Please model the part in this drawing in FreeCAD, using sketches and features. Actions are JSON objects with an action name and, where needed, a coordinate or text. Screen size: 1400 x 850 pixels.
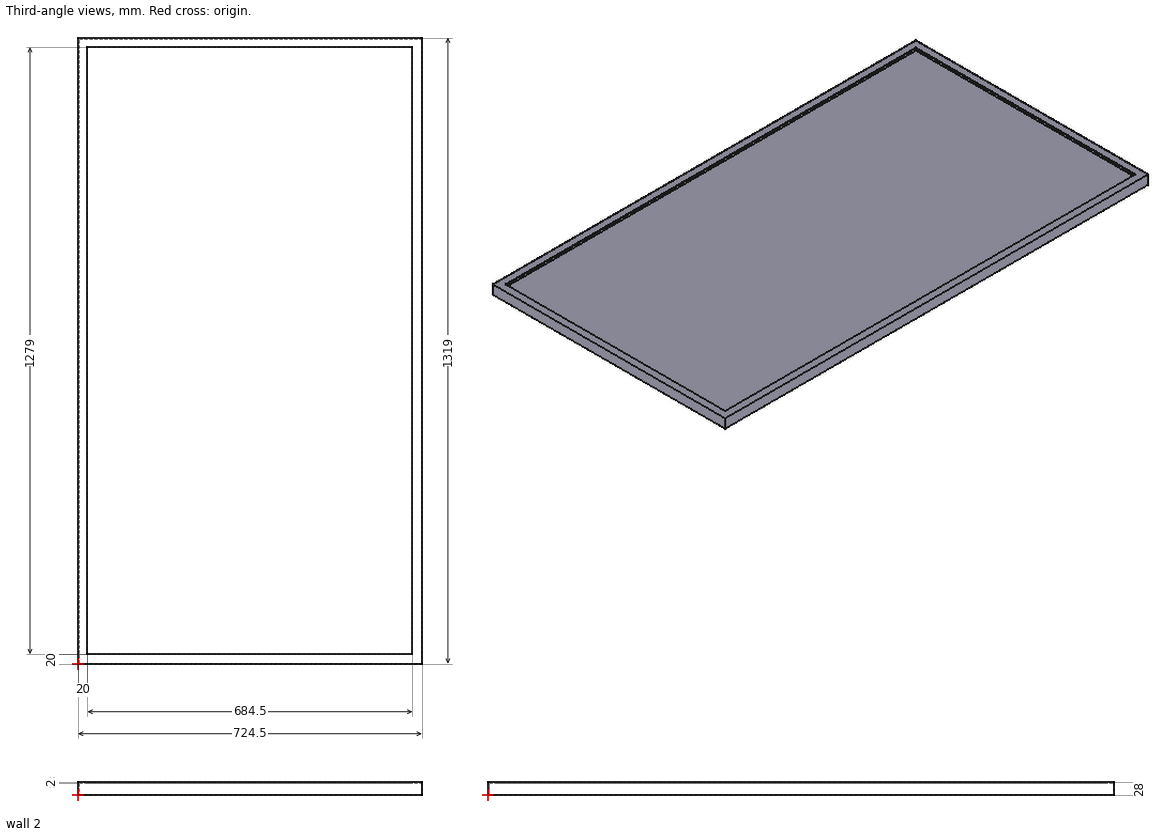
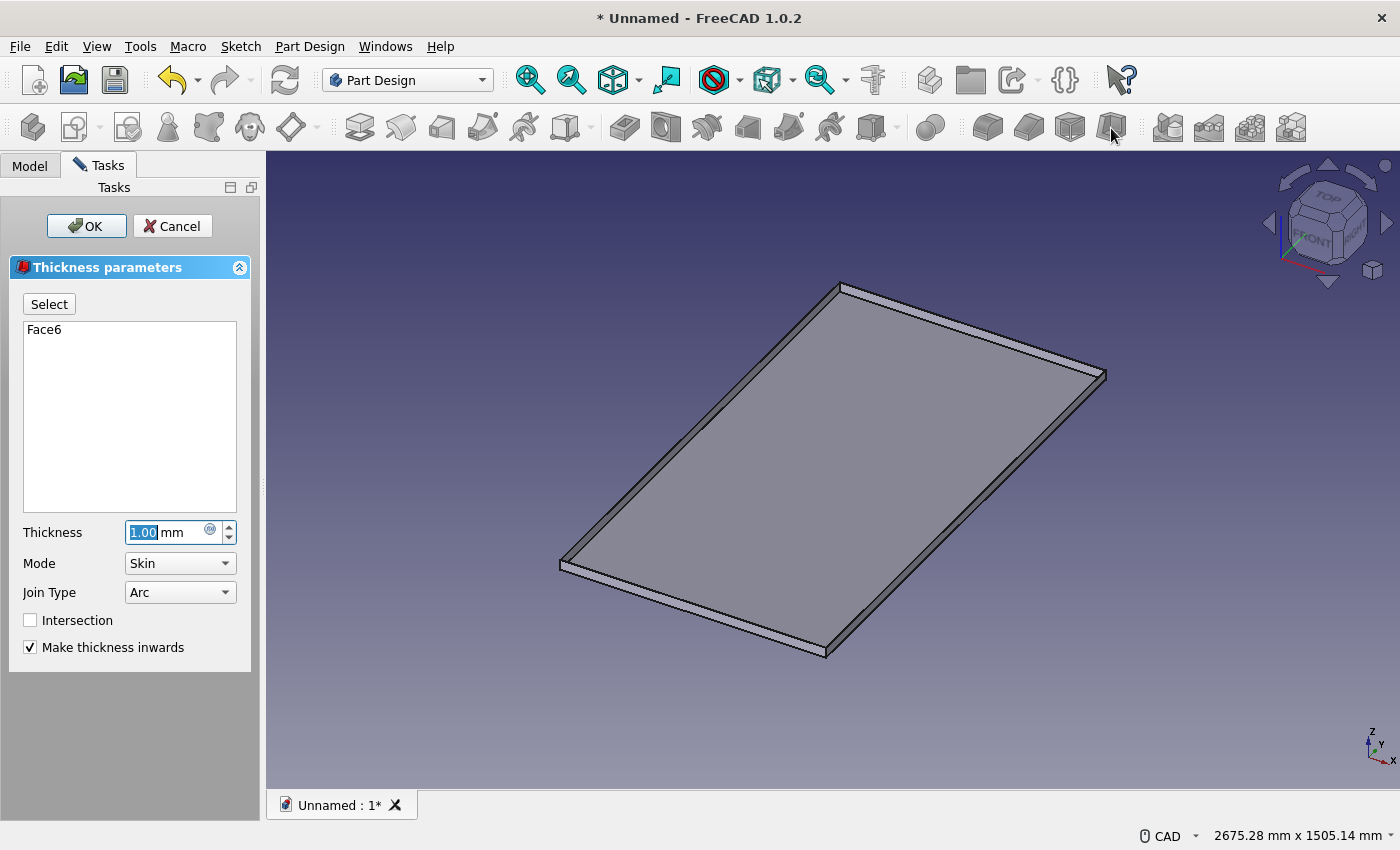
{"action": "type", "text": "2"}
{"action": "key", "text": "Tab"}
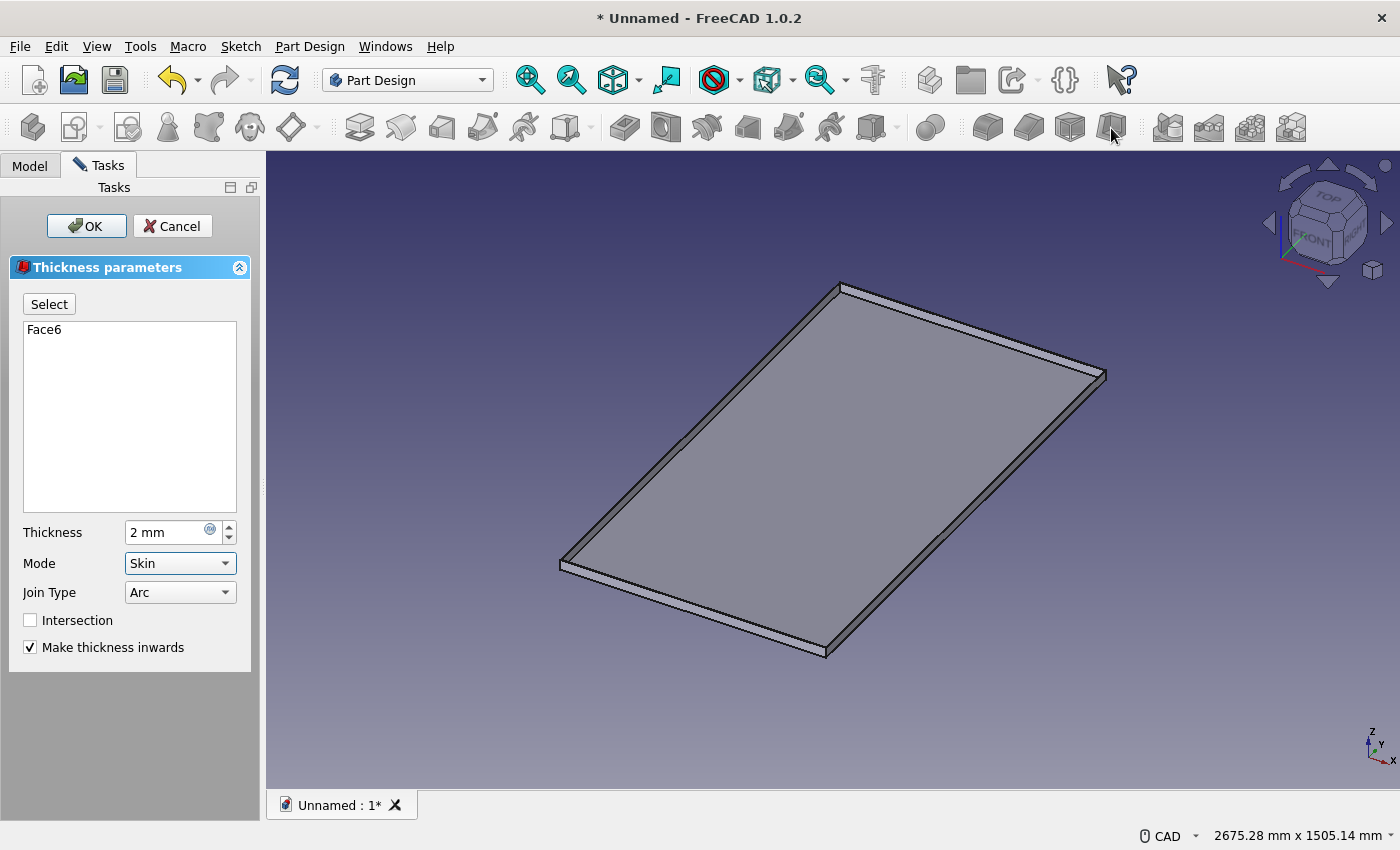
{"action": "left_click", "coordinate": [181, 592]}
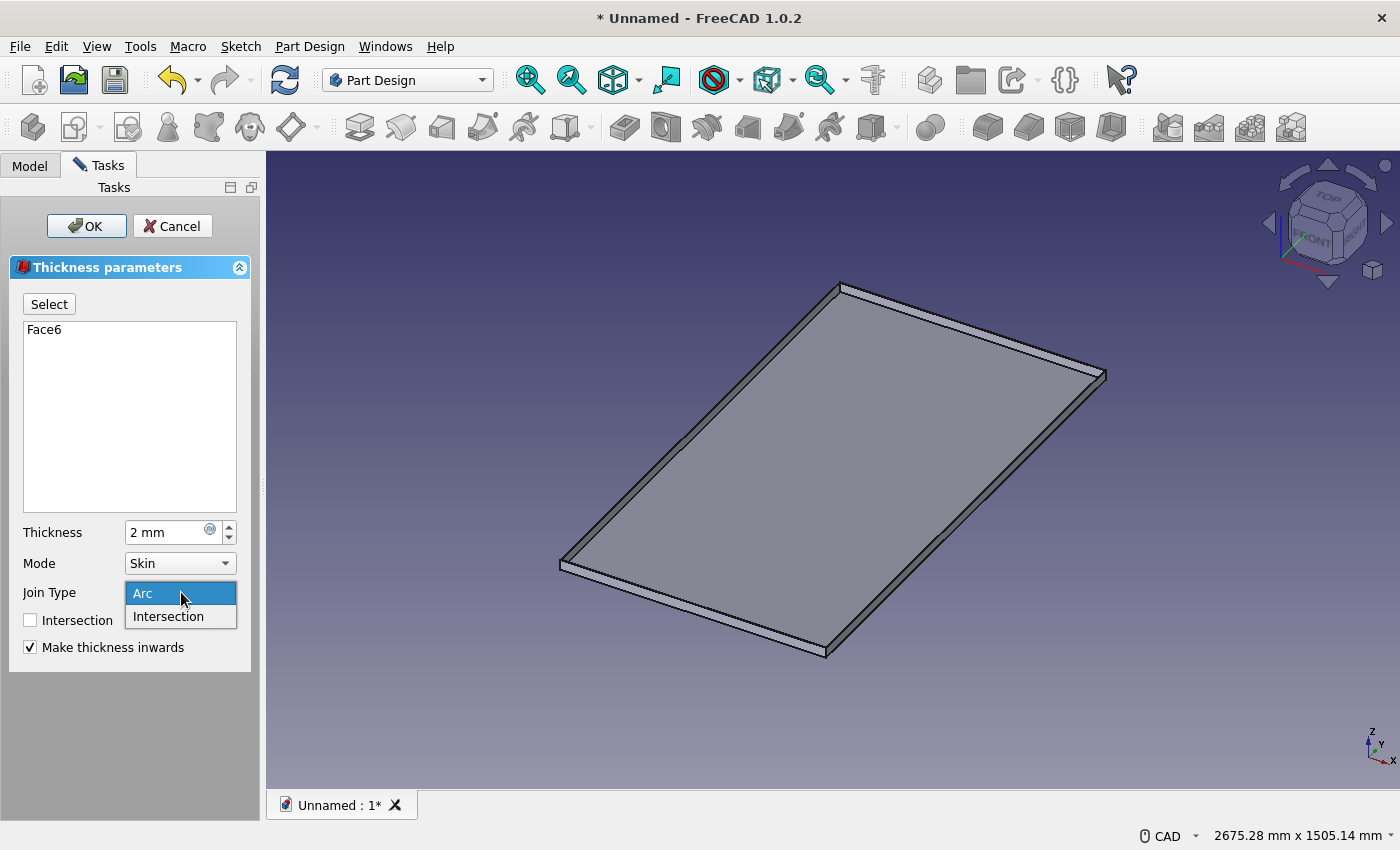
{"action": "left_click", "coordinate": [179, 616]}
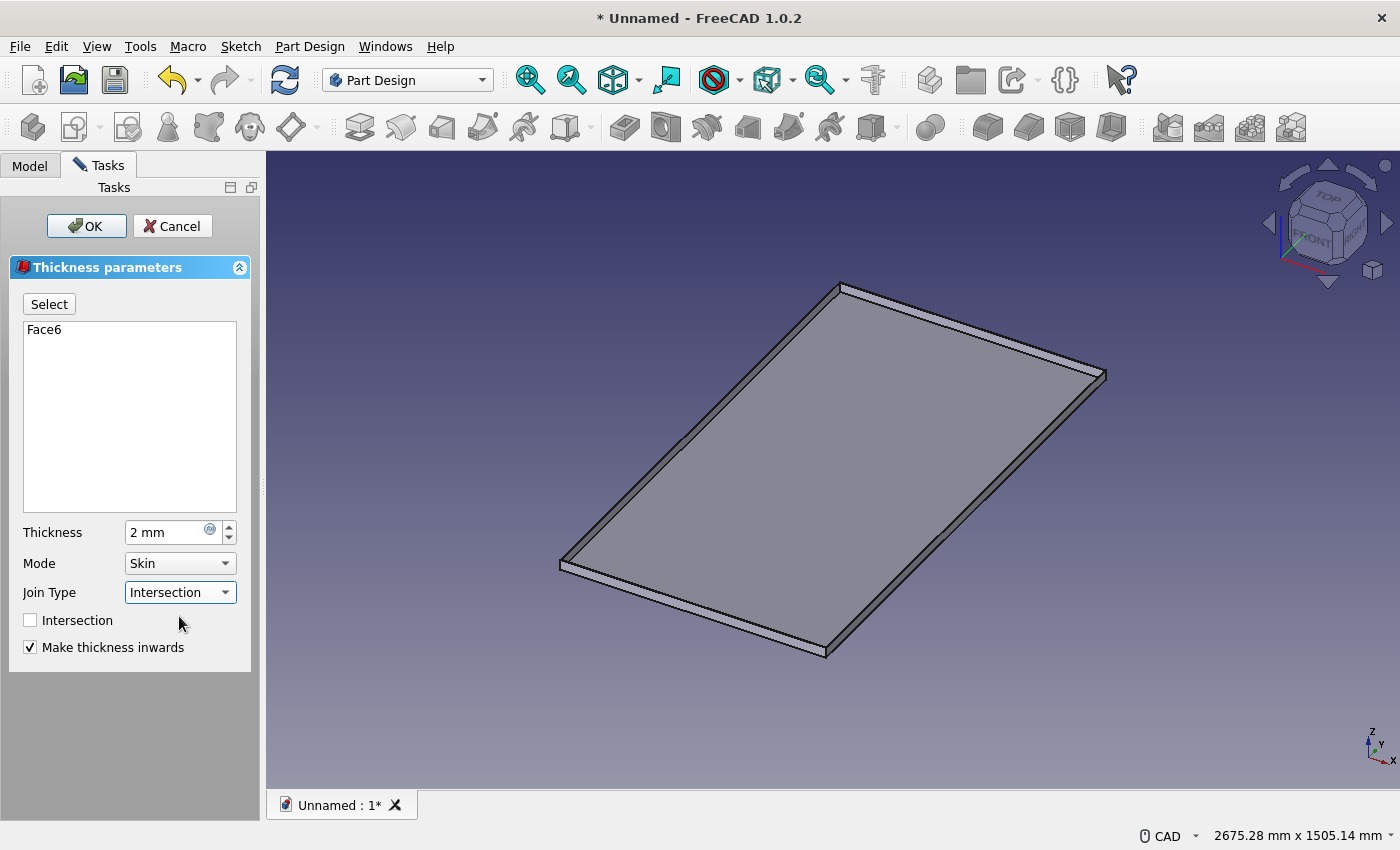
{"action": "left_click", "coordinate": [87, 226]}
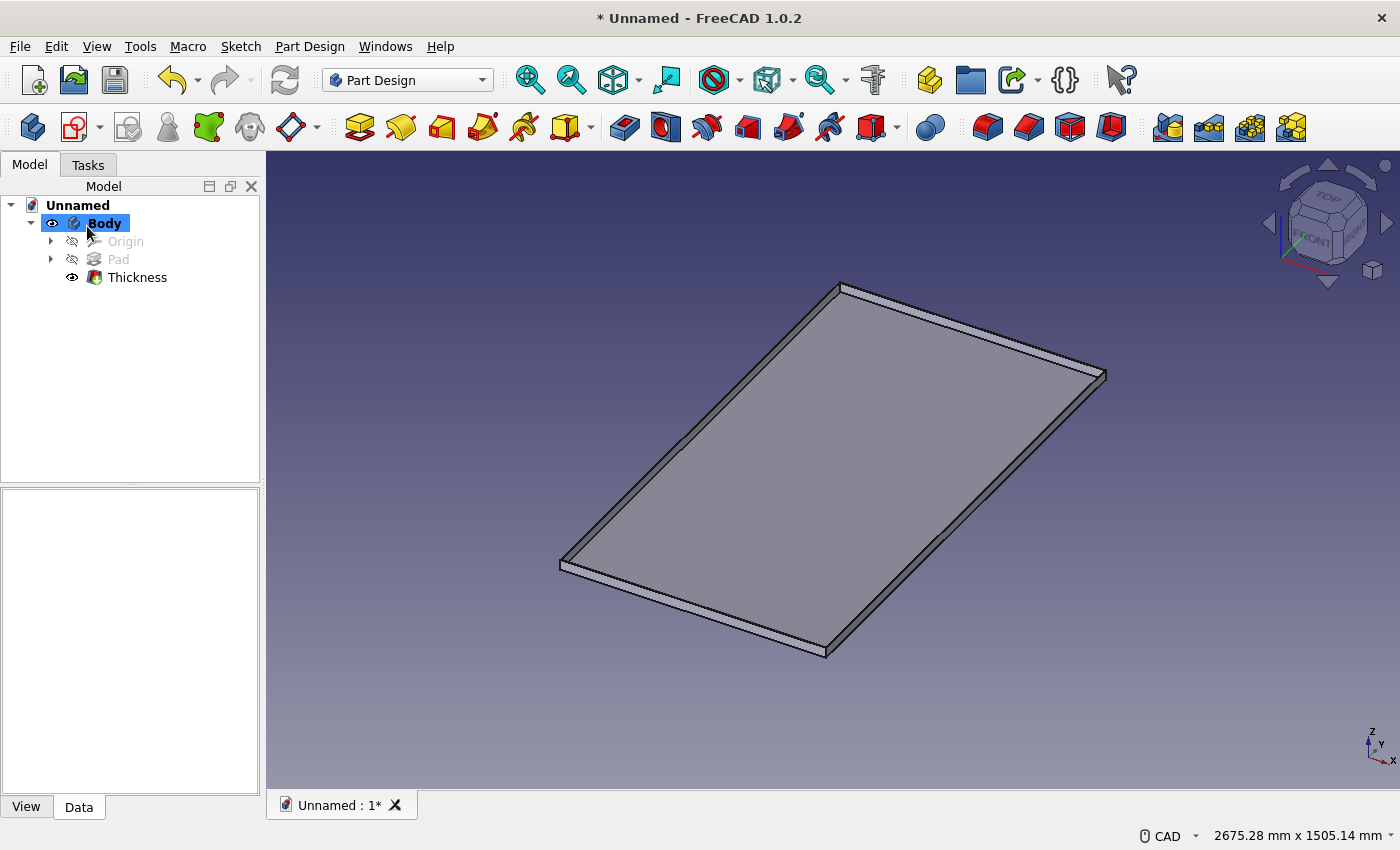
{"action": "scroll", "coordinate": [1017, 340], "scroll_direction": "up", "scroll_amount": 15}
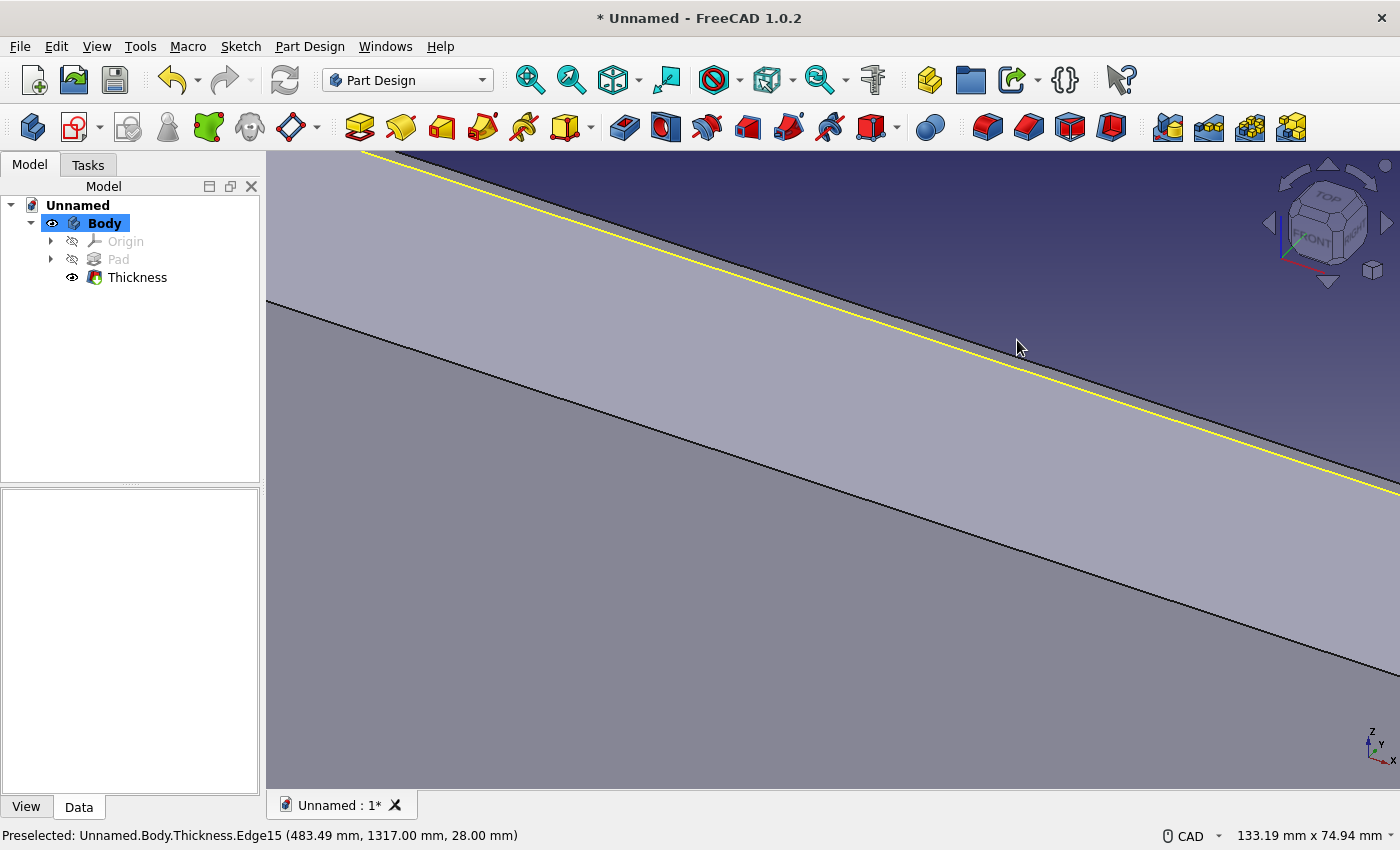
{"action": "scroll", "coordinate": [1001, 358], "scroll_direction": "up", "scroll_amount": 4}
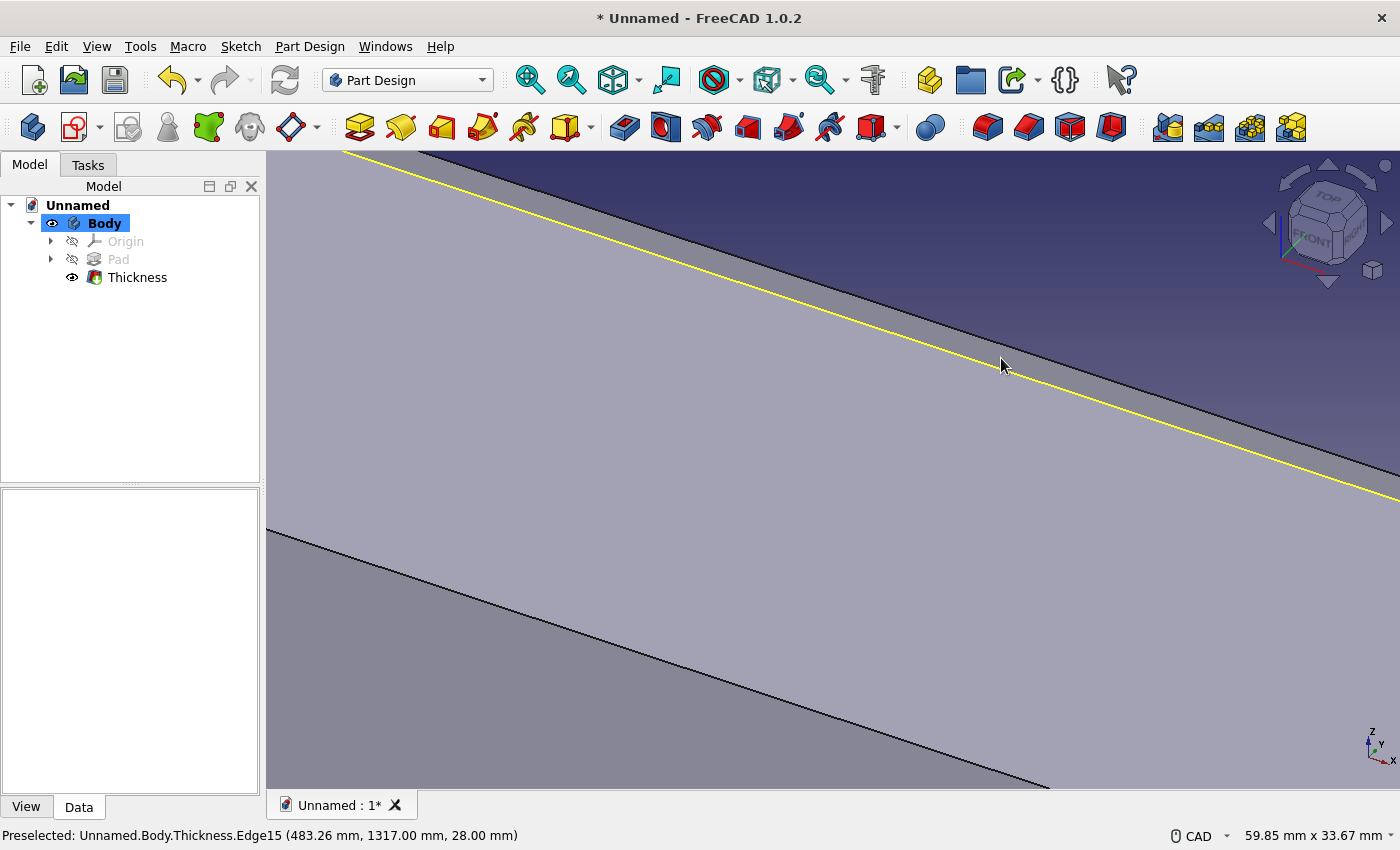
{"action": "left_click", "coordinate": [531, 80]}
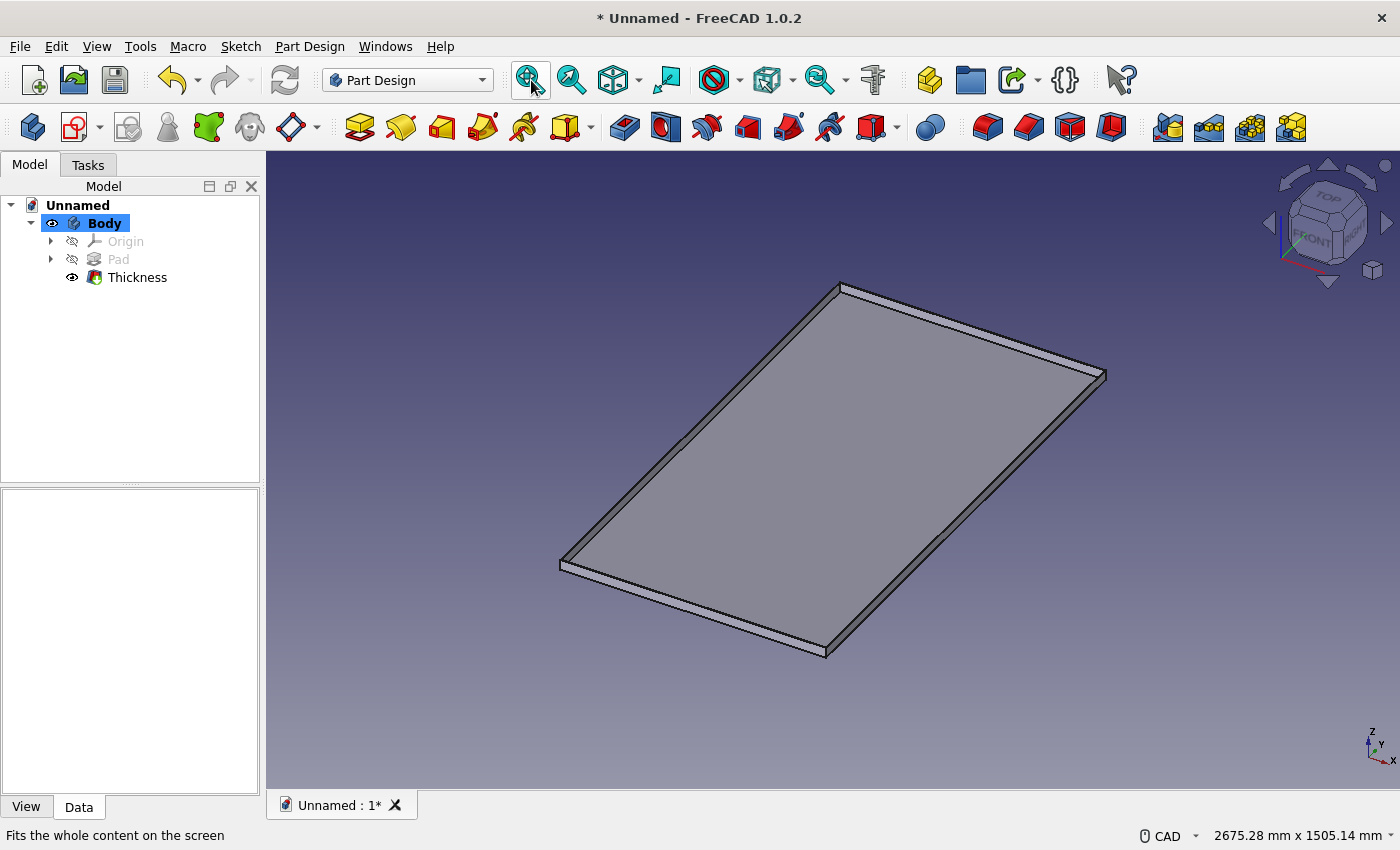
{"action": "key", "text": "0"}